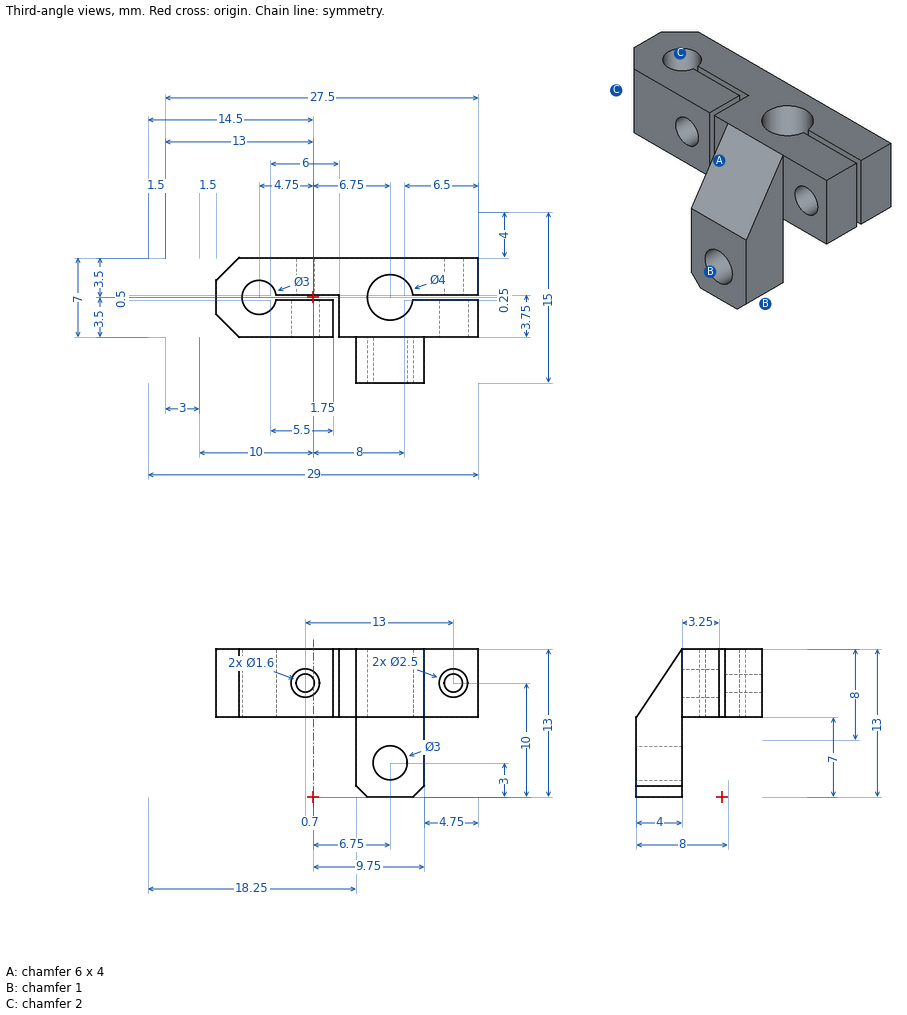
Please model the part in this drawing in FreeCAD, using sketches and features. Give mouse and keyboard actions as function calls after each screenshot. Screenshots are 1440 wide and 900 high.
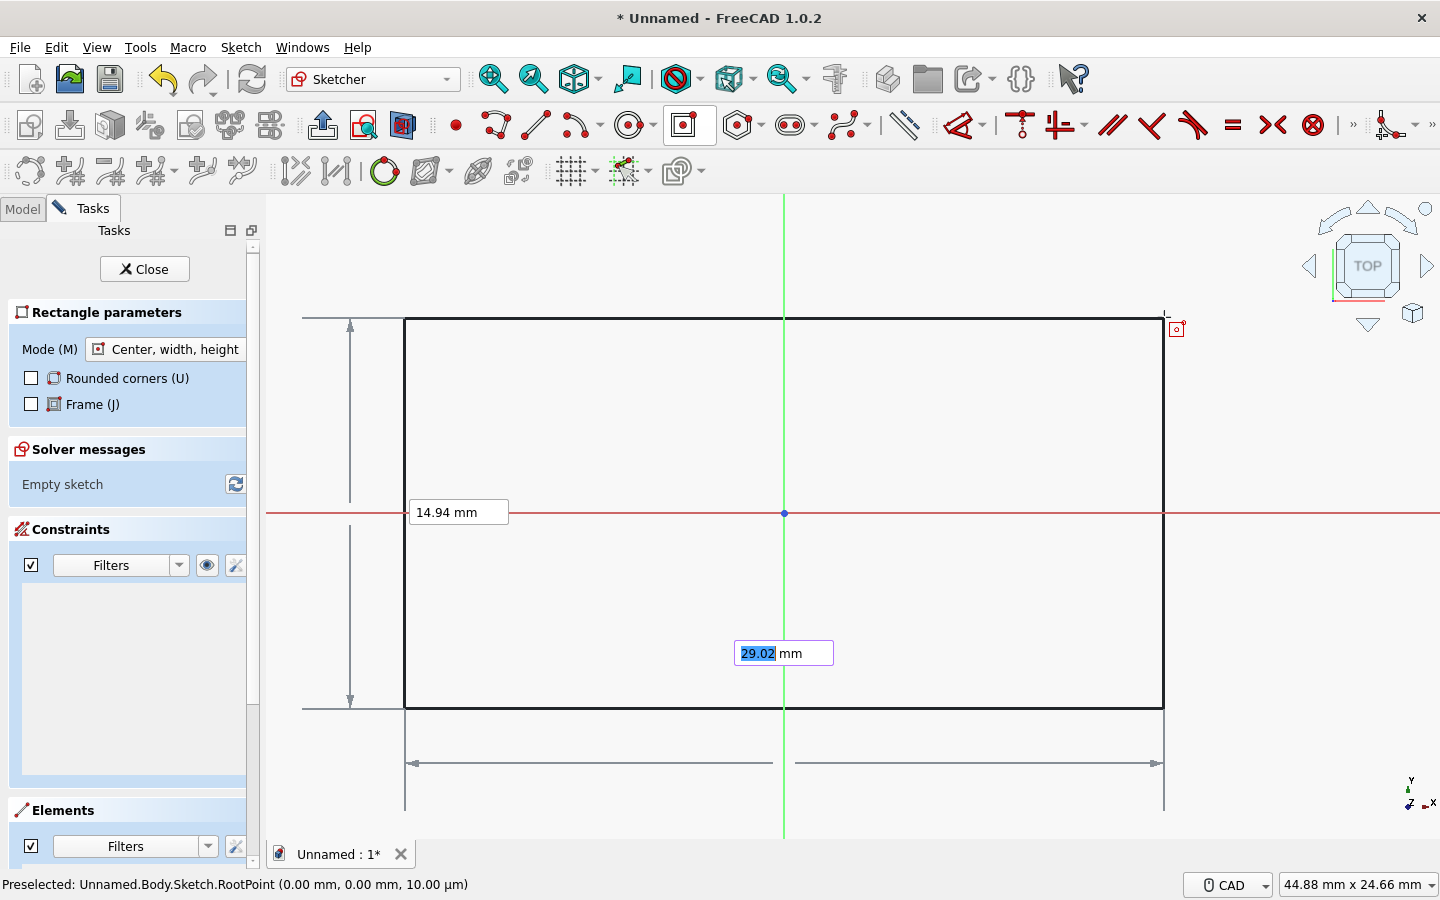
text(29)
key(Tab)
text(15)
key(Return)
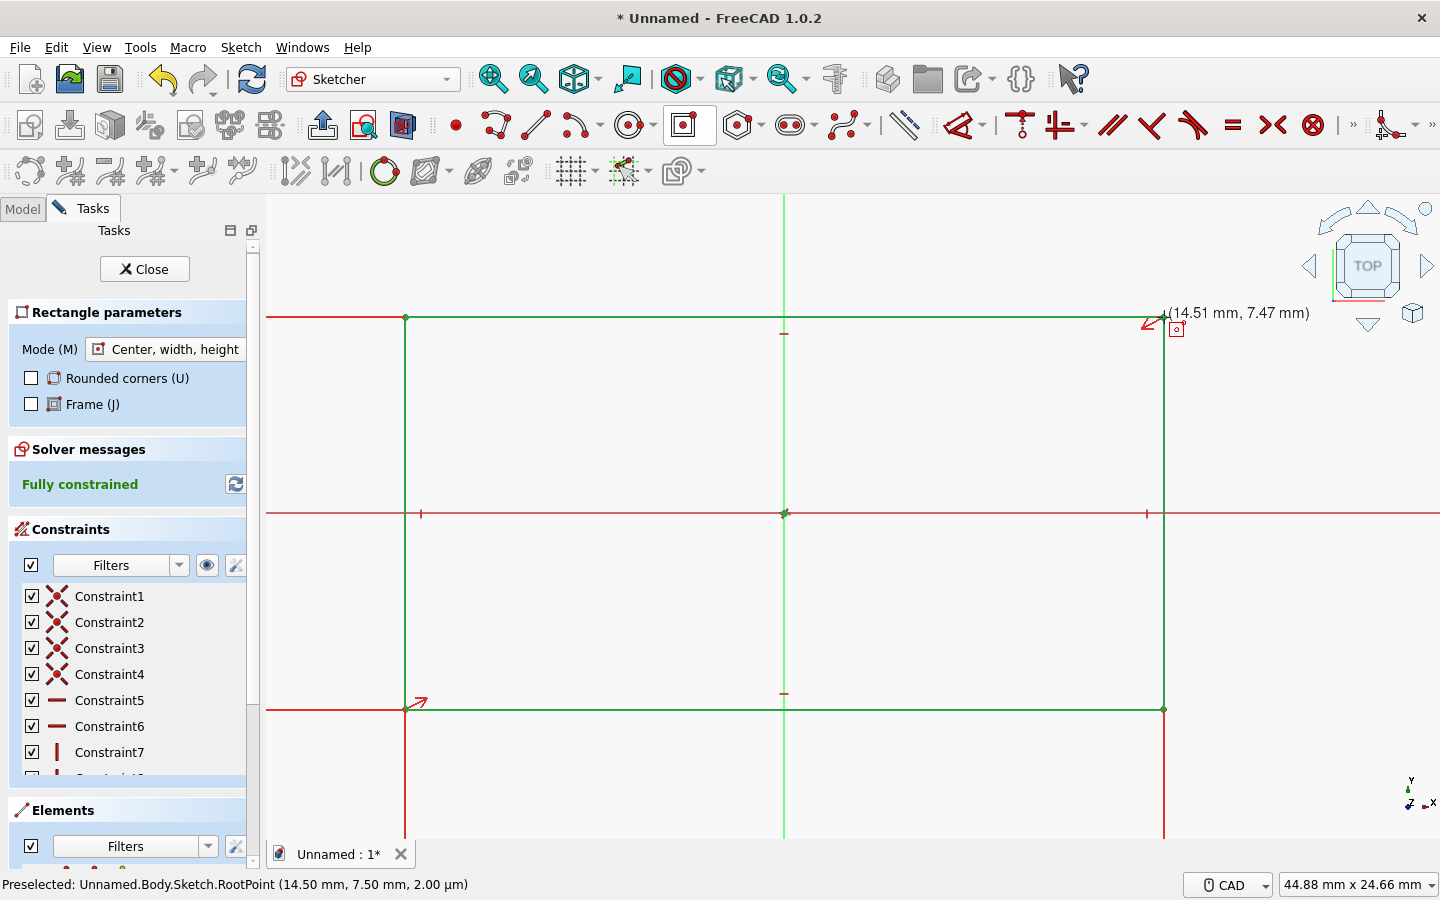
click(630, 126)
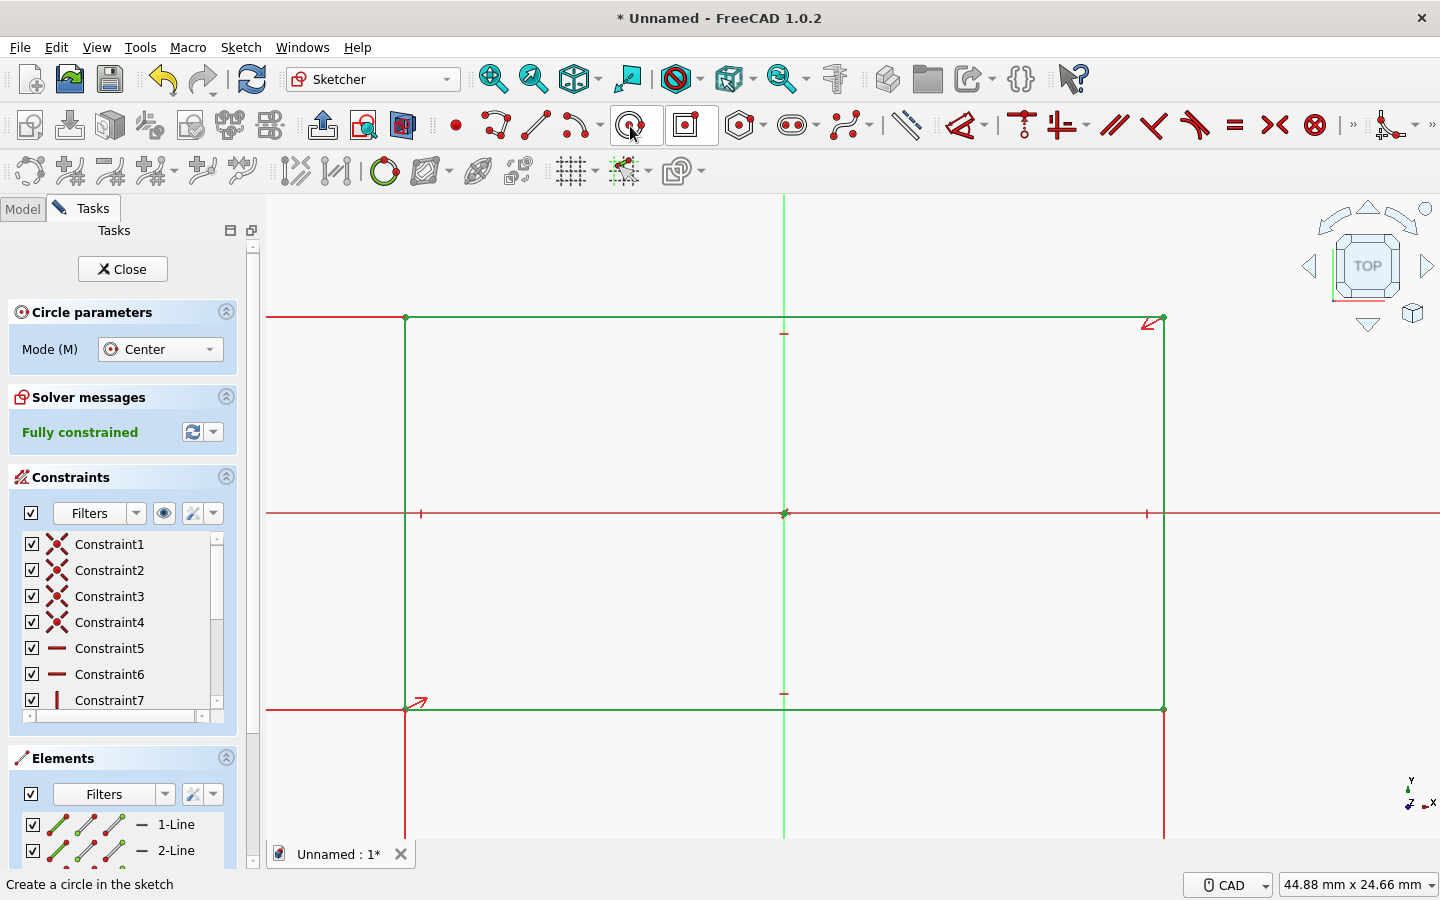
click(660, 513)
move(688, 486)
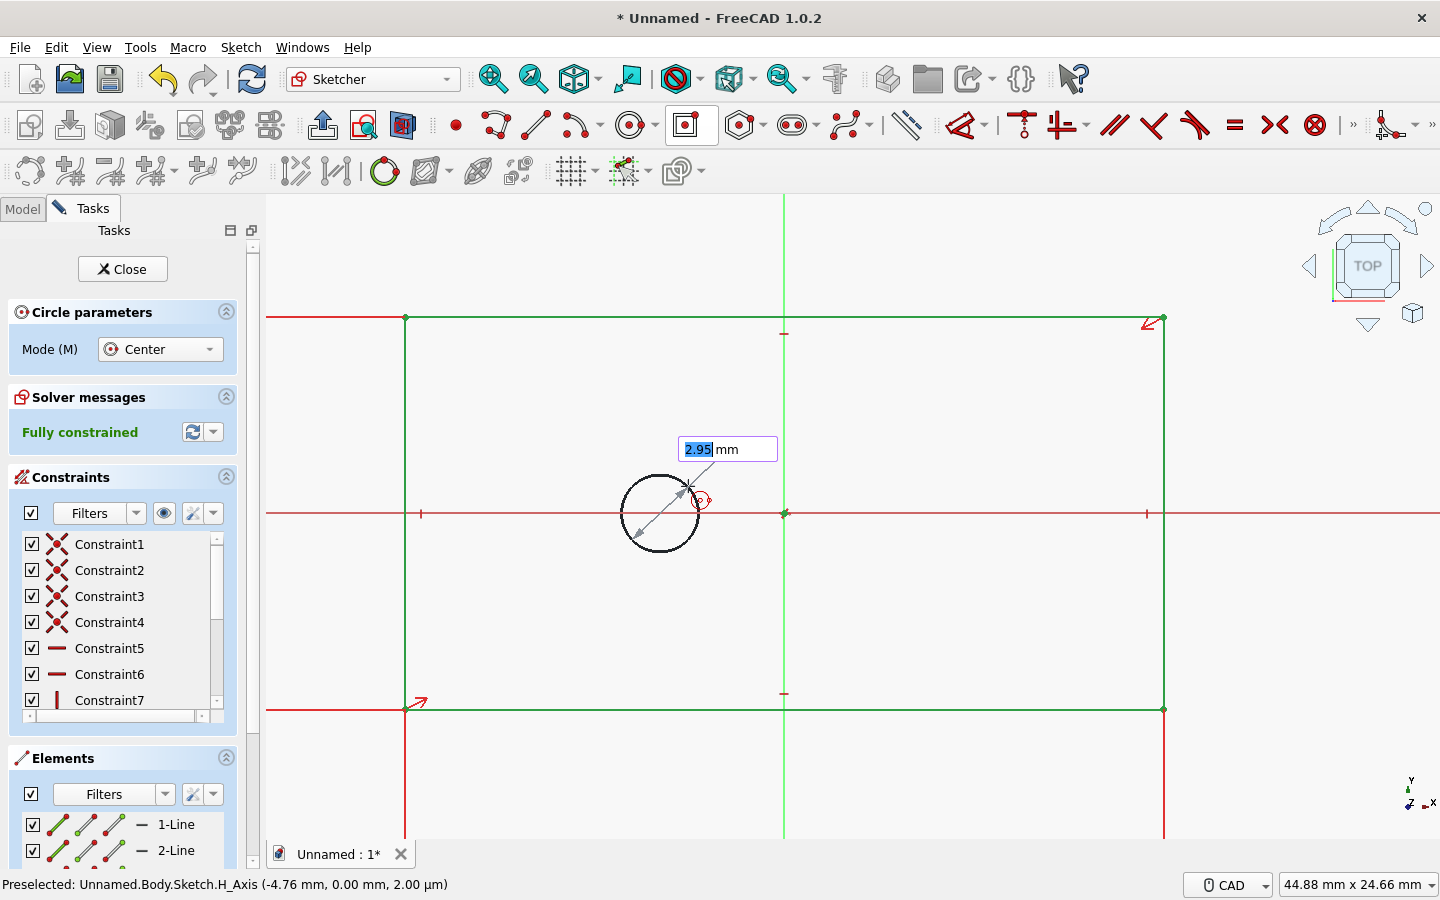
text(3)
key(Return)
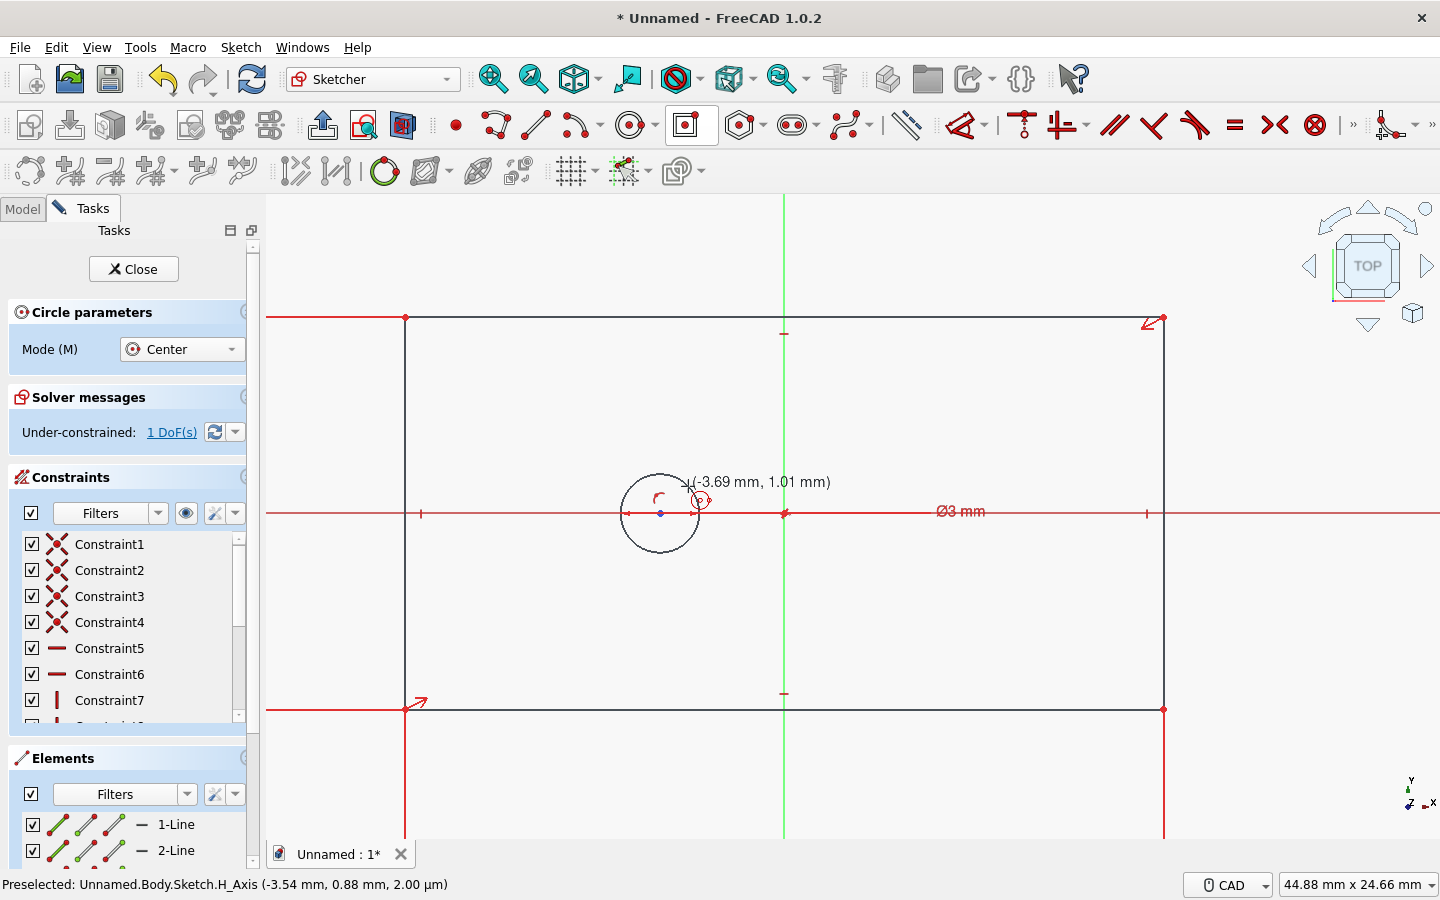
click(961, 513)
move(998, 476)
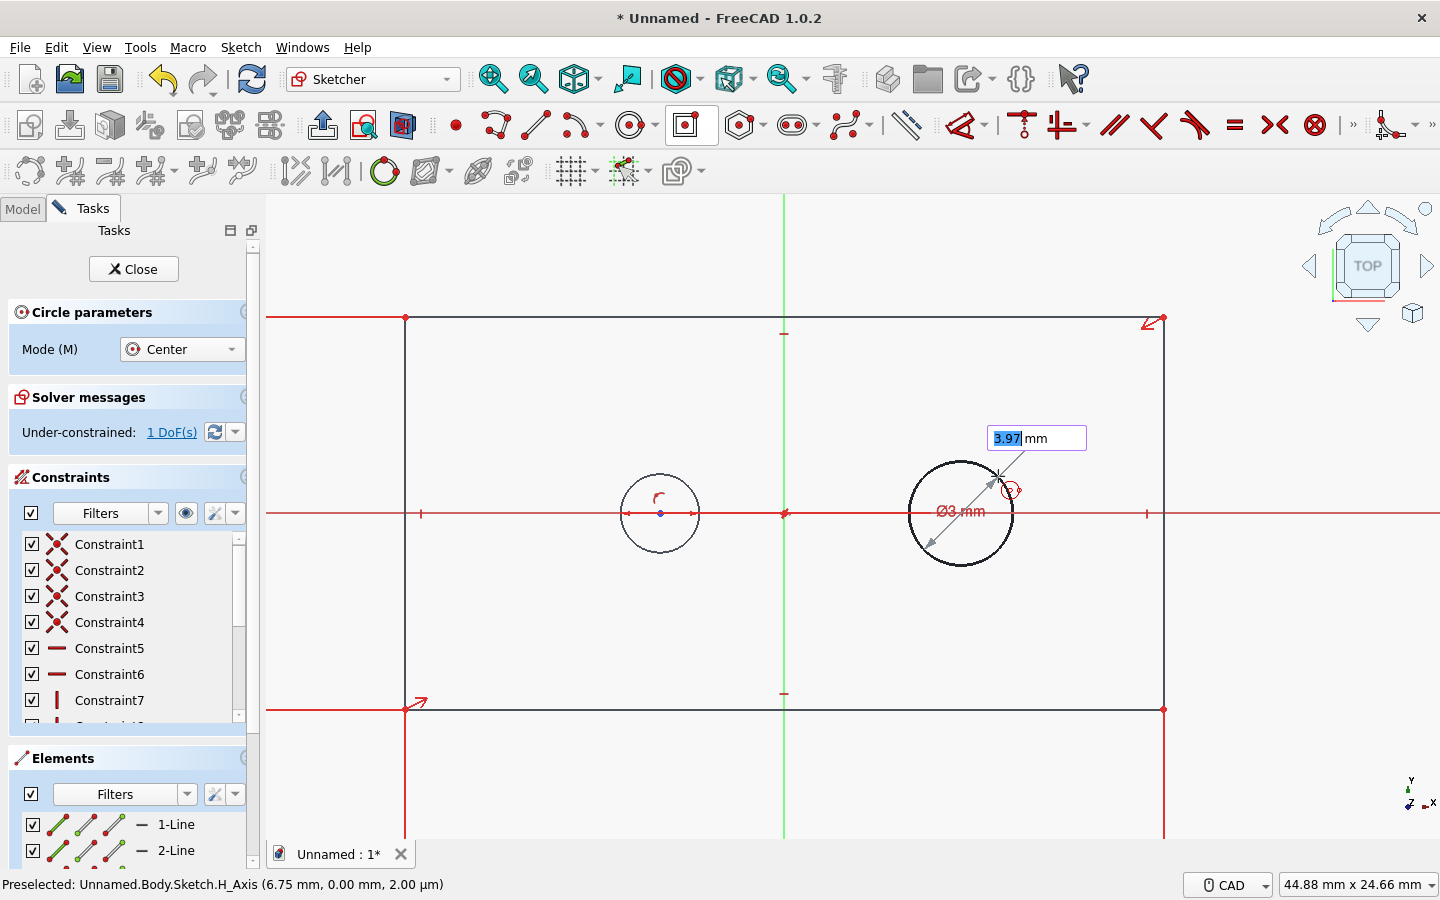
text(4)
key(Return)
key(Escape)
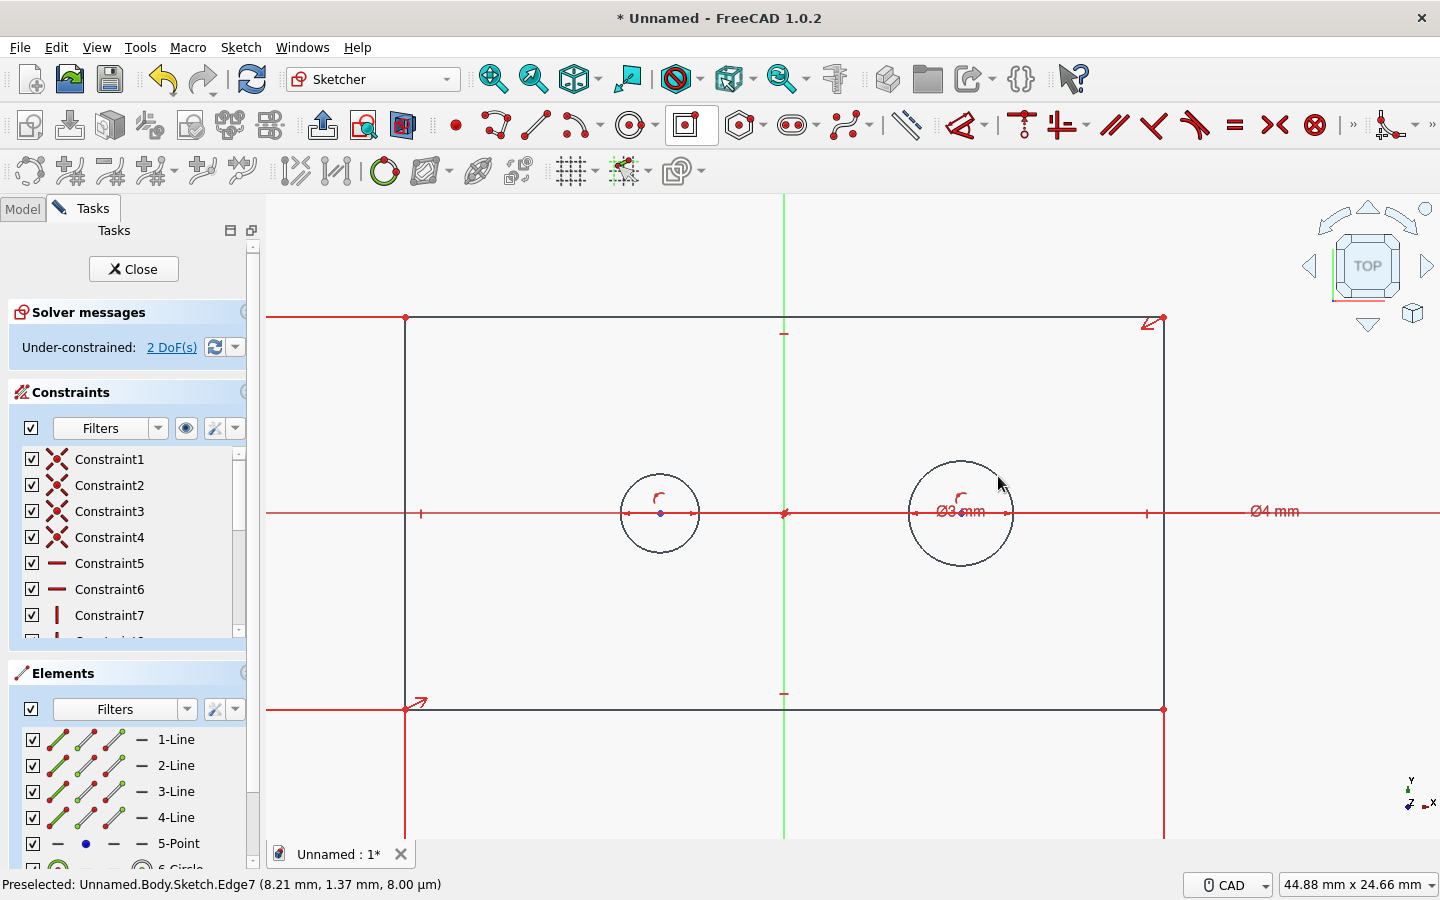
click(960, 126)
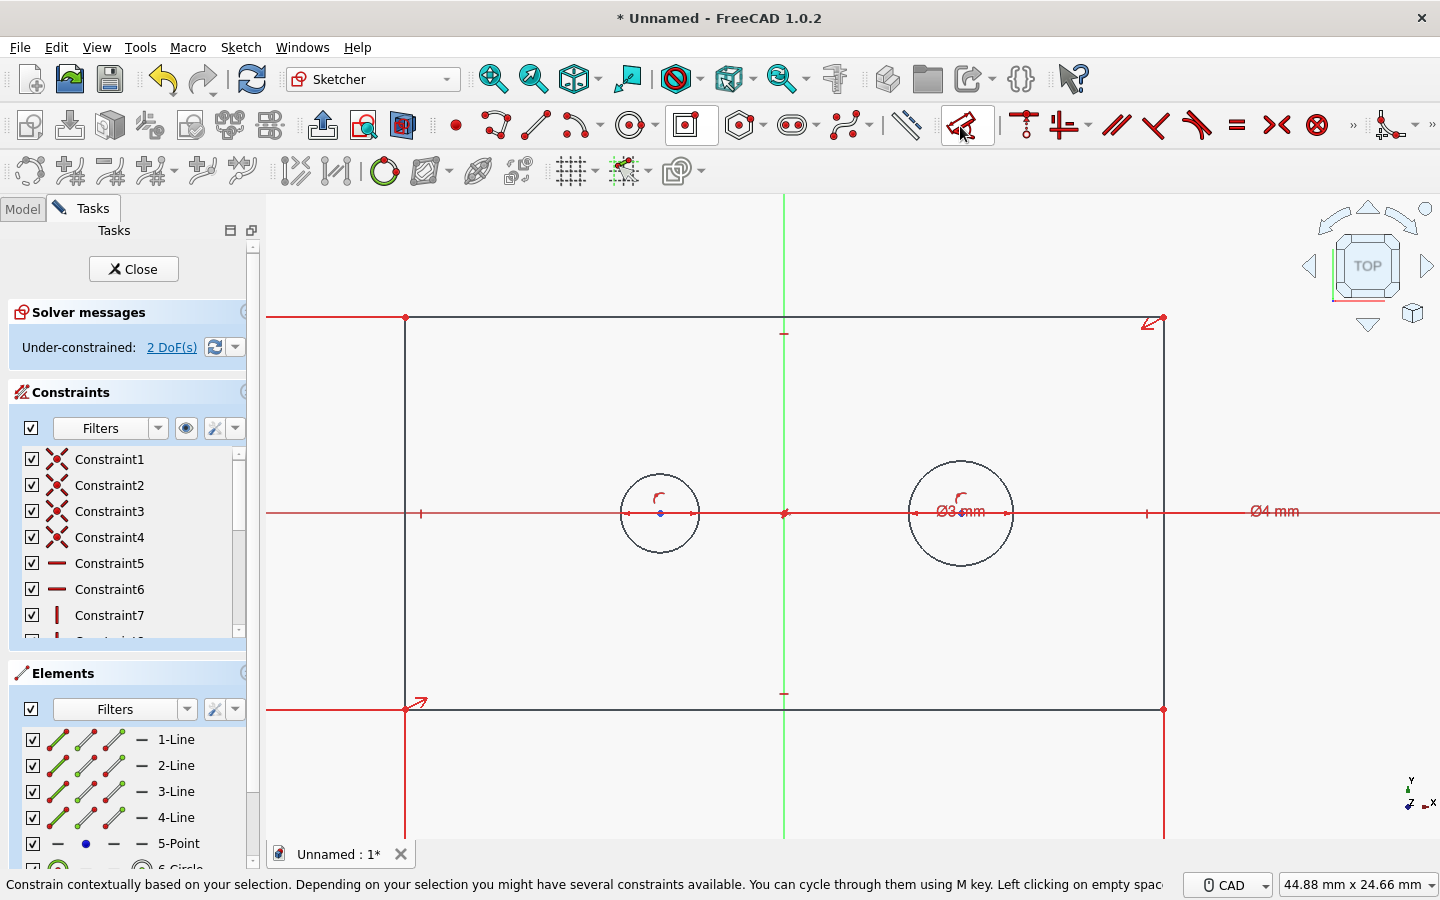
click(660, 513)
click(722, 547)